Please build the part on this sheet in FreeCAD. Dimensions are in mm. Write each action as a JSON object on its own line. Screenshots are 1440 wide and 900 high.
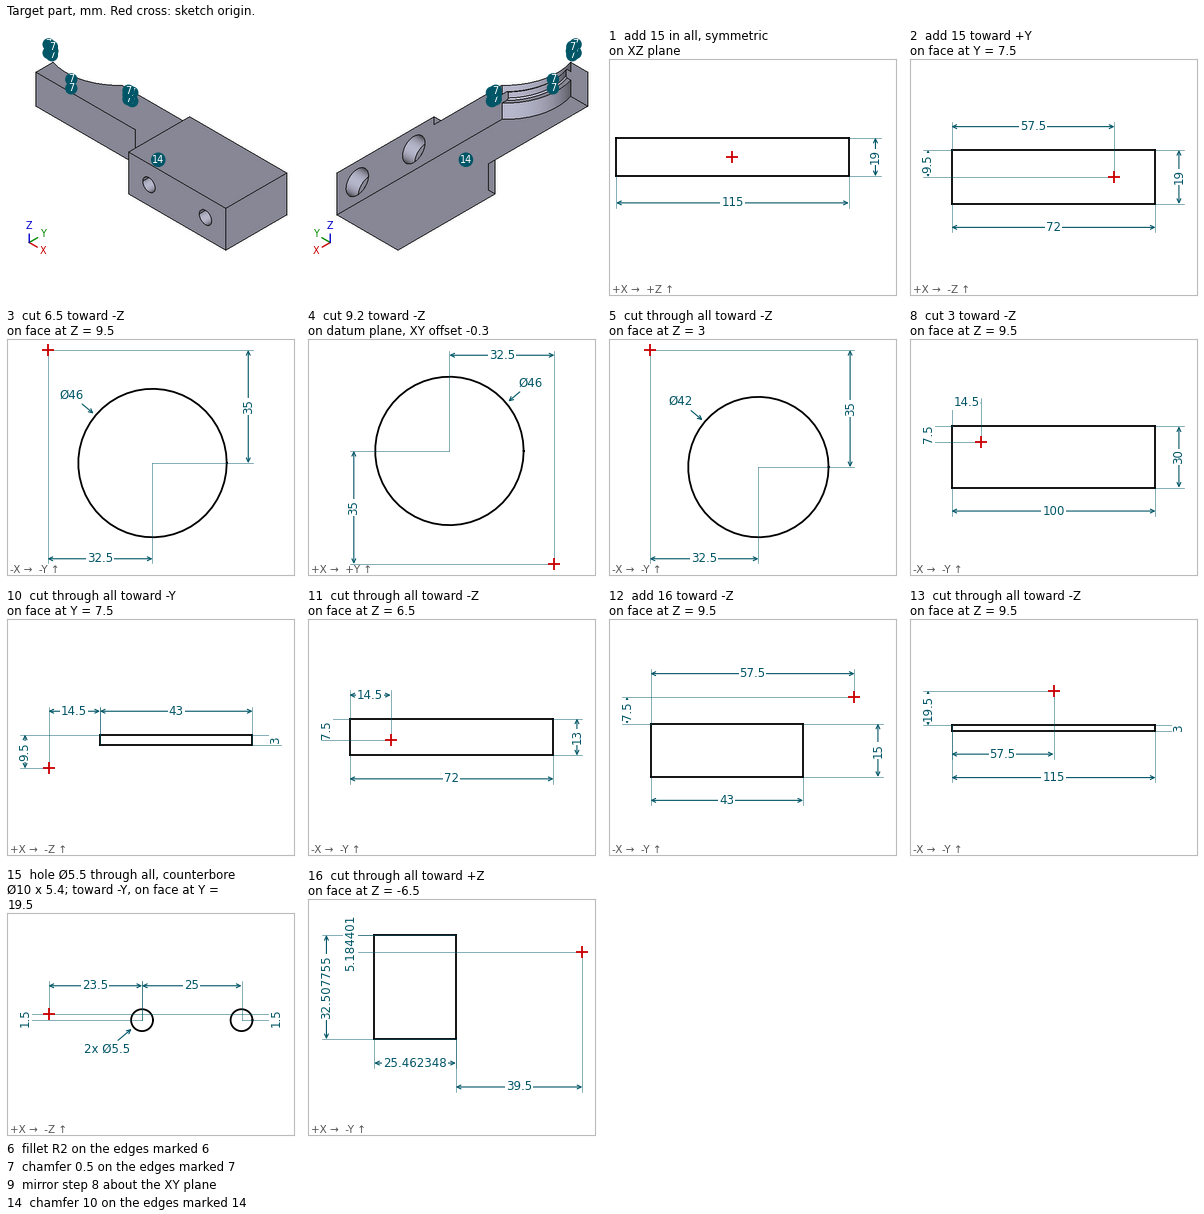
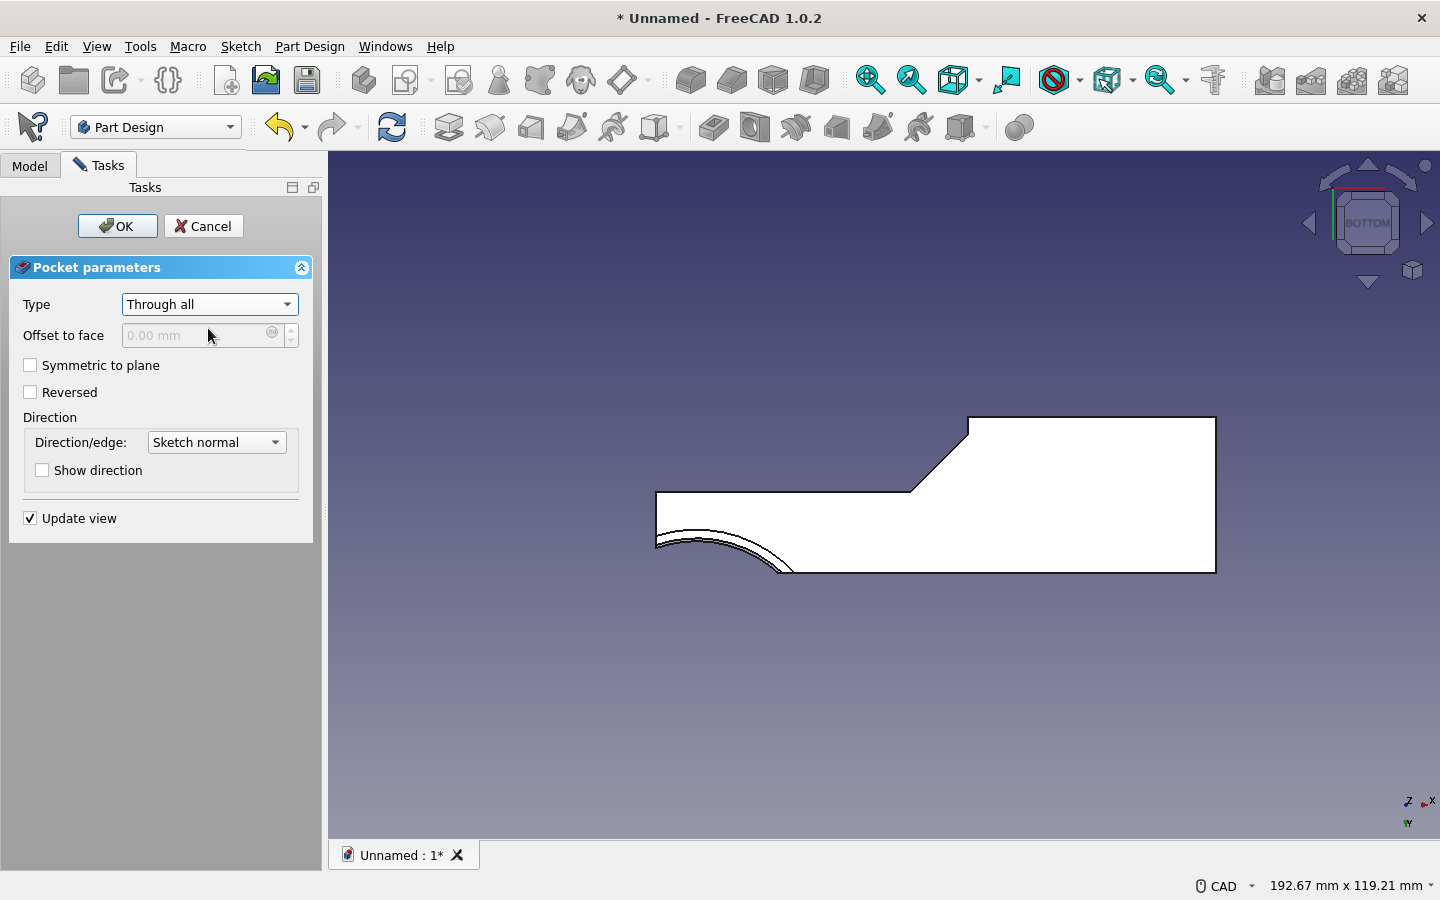
{"action": "left_click", "coordinate": [118, 226]}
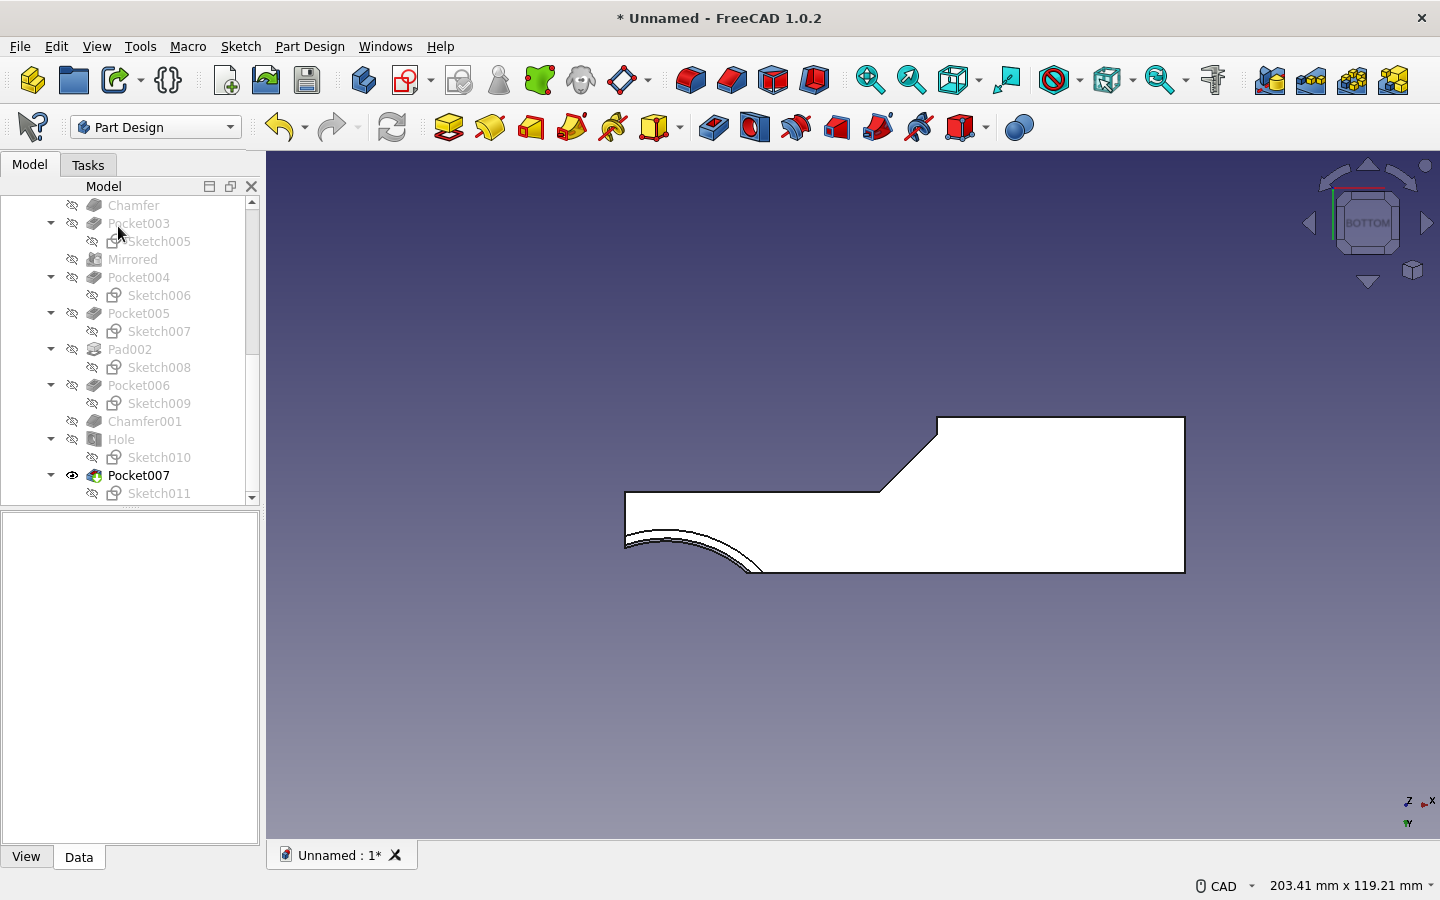
{"action": "key", "text": "0"}